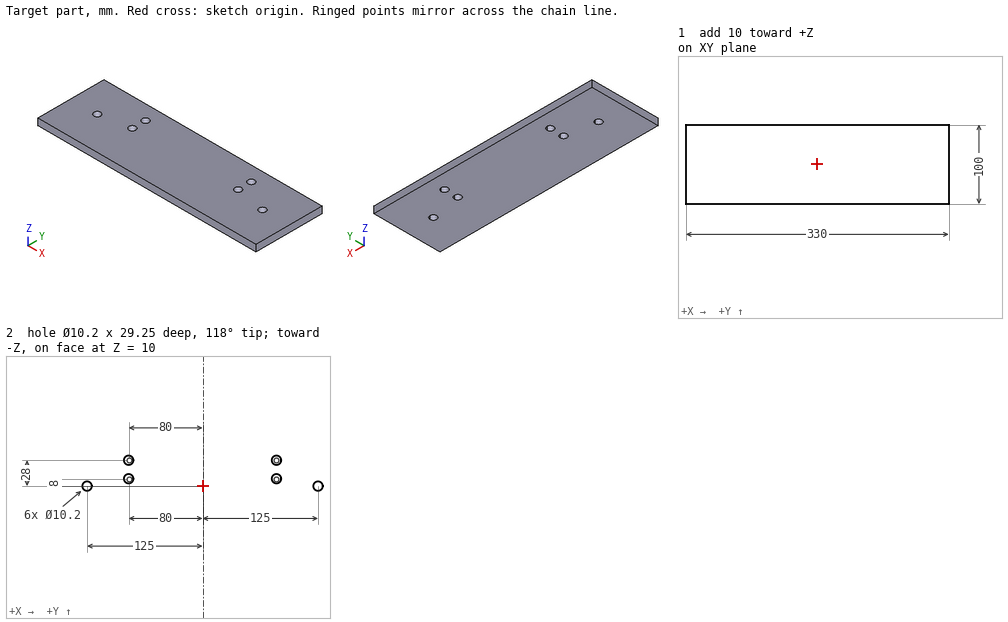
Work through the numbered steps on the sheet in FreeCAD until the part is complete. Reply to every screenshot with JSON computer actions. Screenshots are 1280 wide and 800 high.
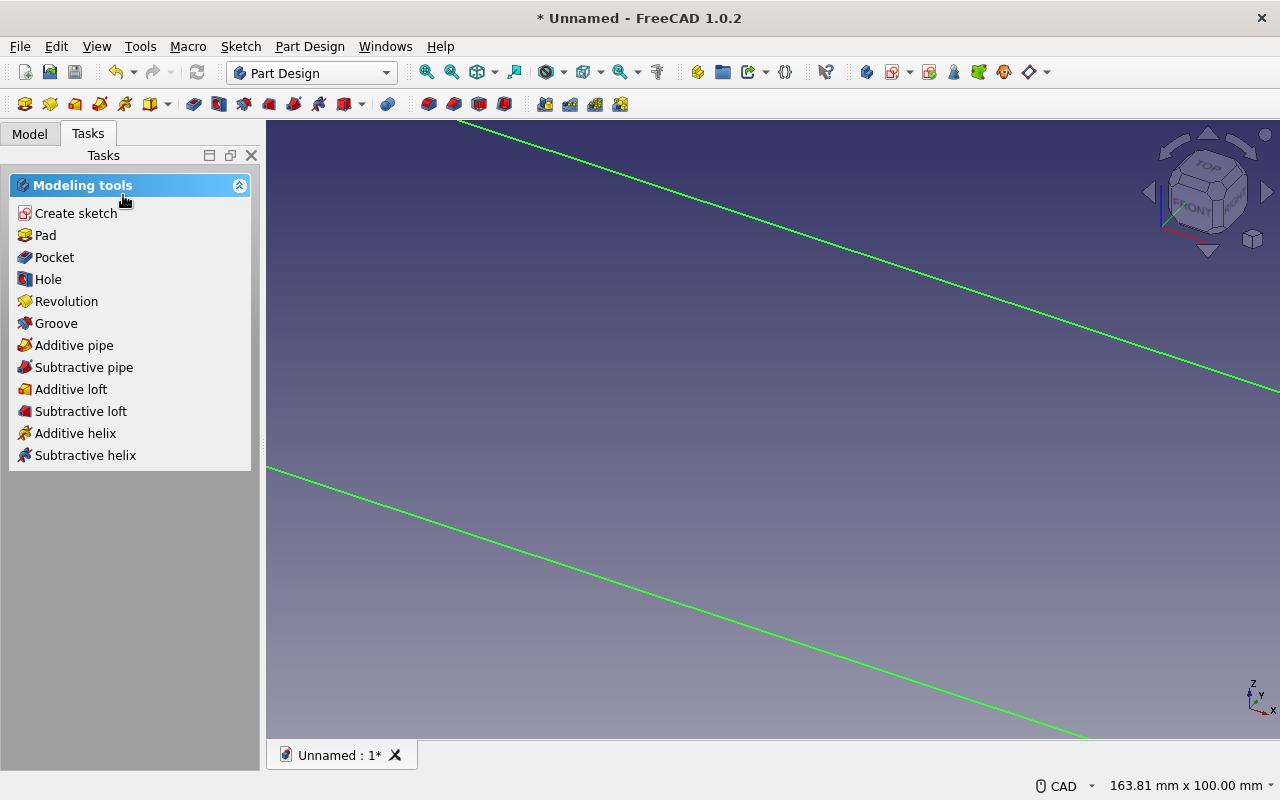
{"action": "left_click", "coordinate": [25, 104]}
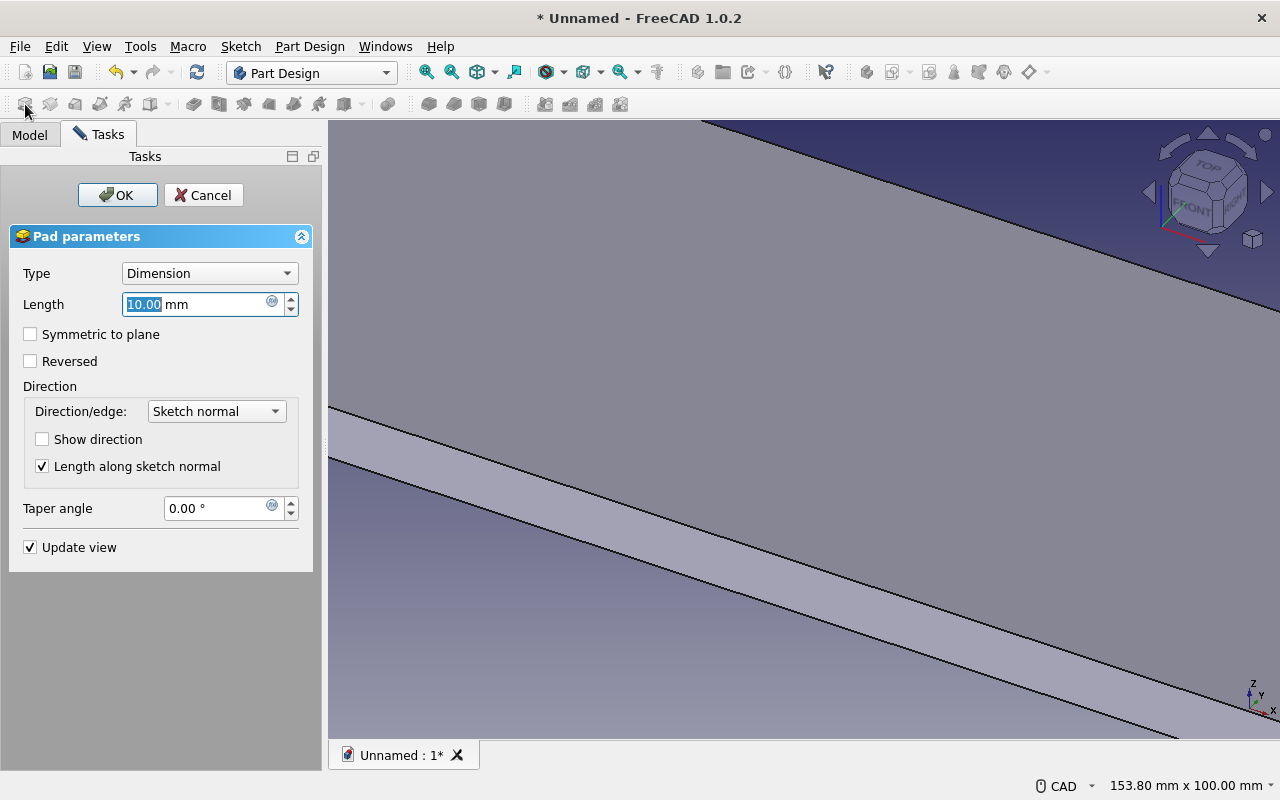
{"action": "type", "text": "10"}
{"action": "key", "text": "Tab"}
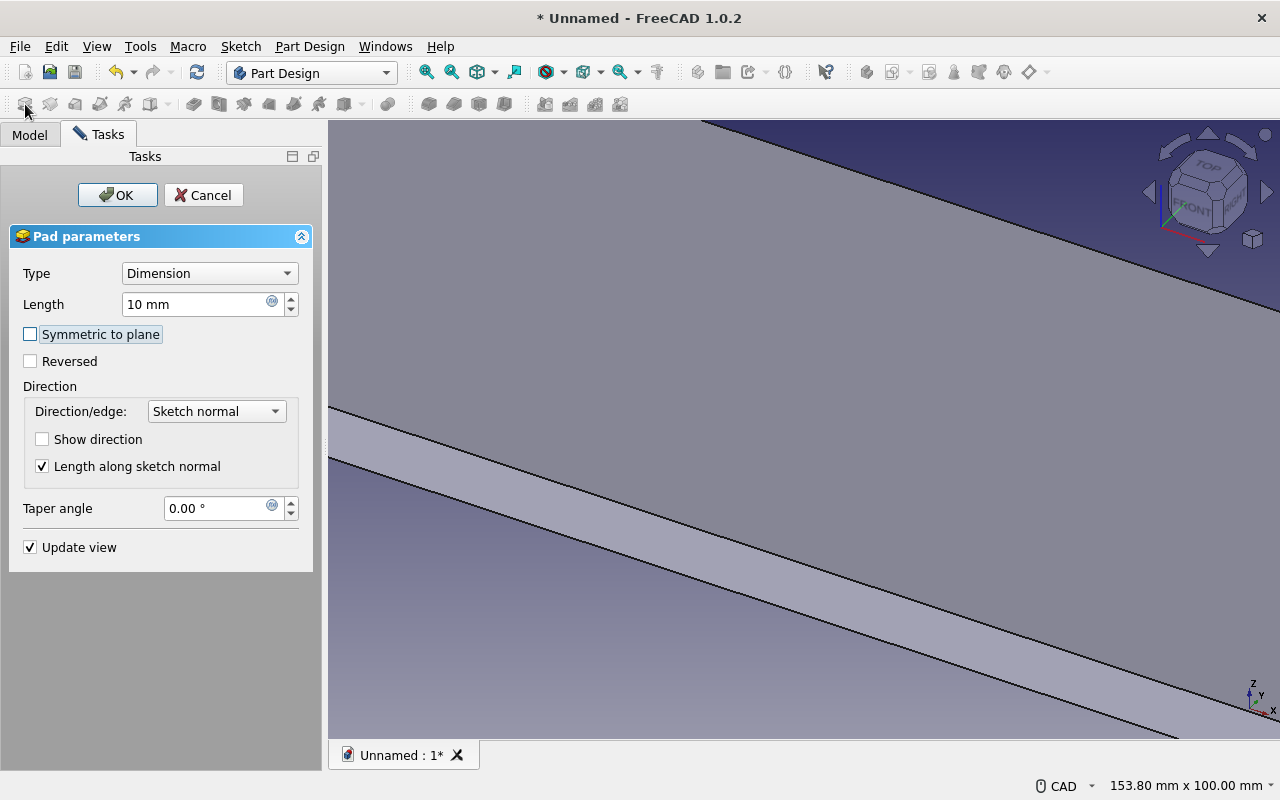
{"action": "left_click", "coordinate": [118, 195]}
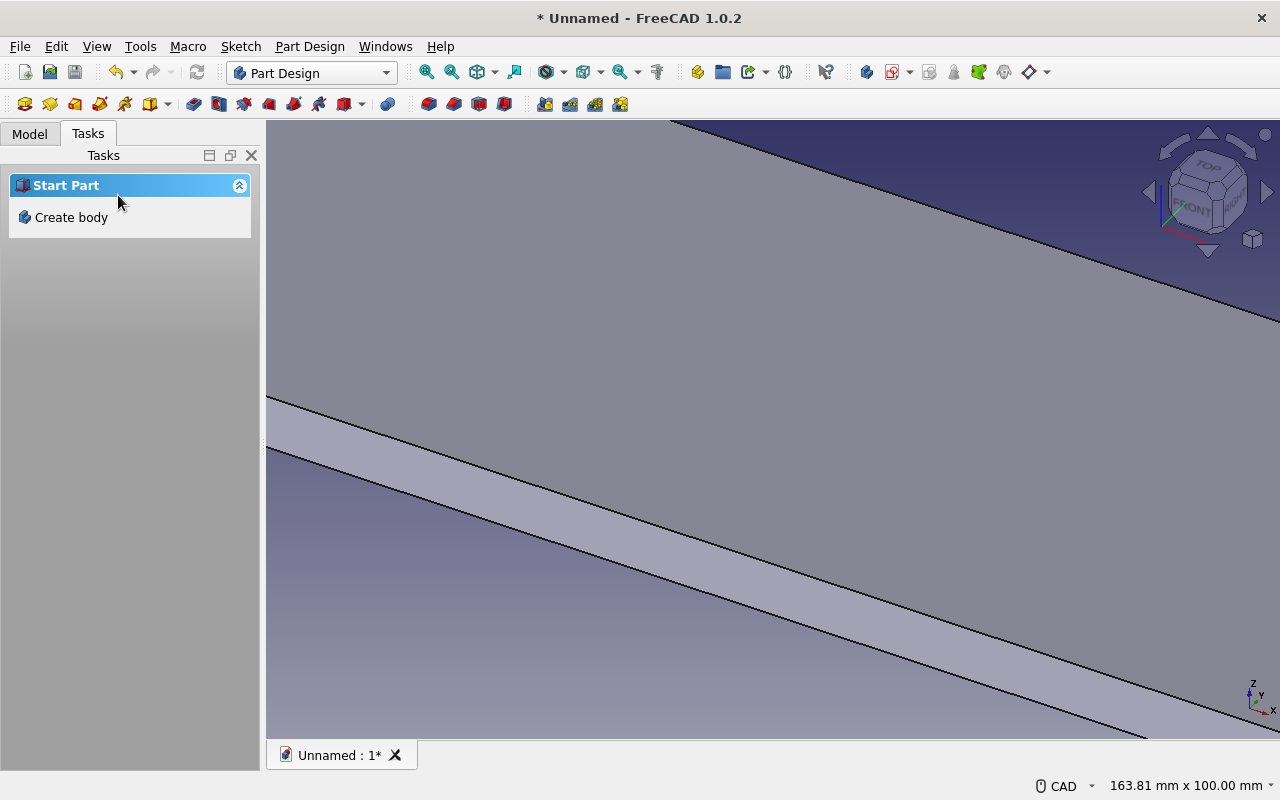
{"action": "left_click", "coordinate": [427, 72]}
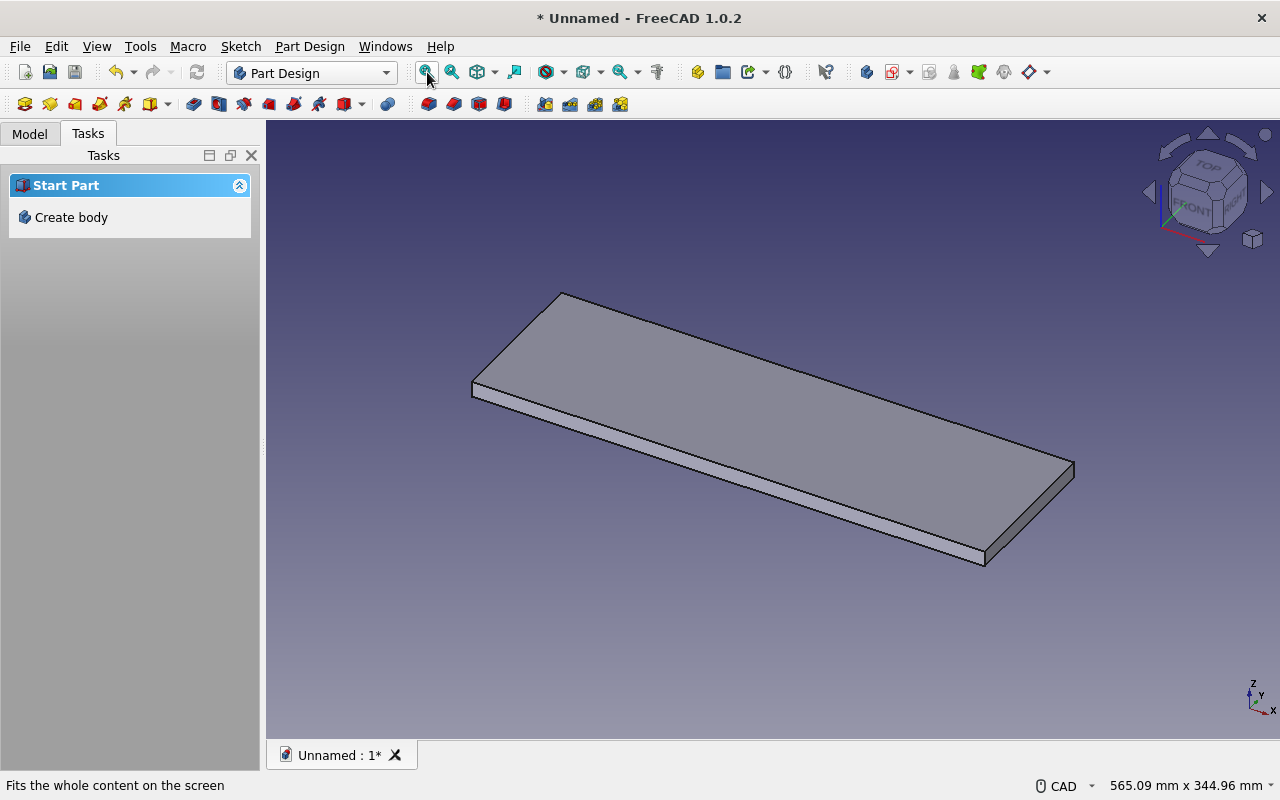
{"action": "left_click", "coordinate": [920, 470]}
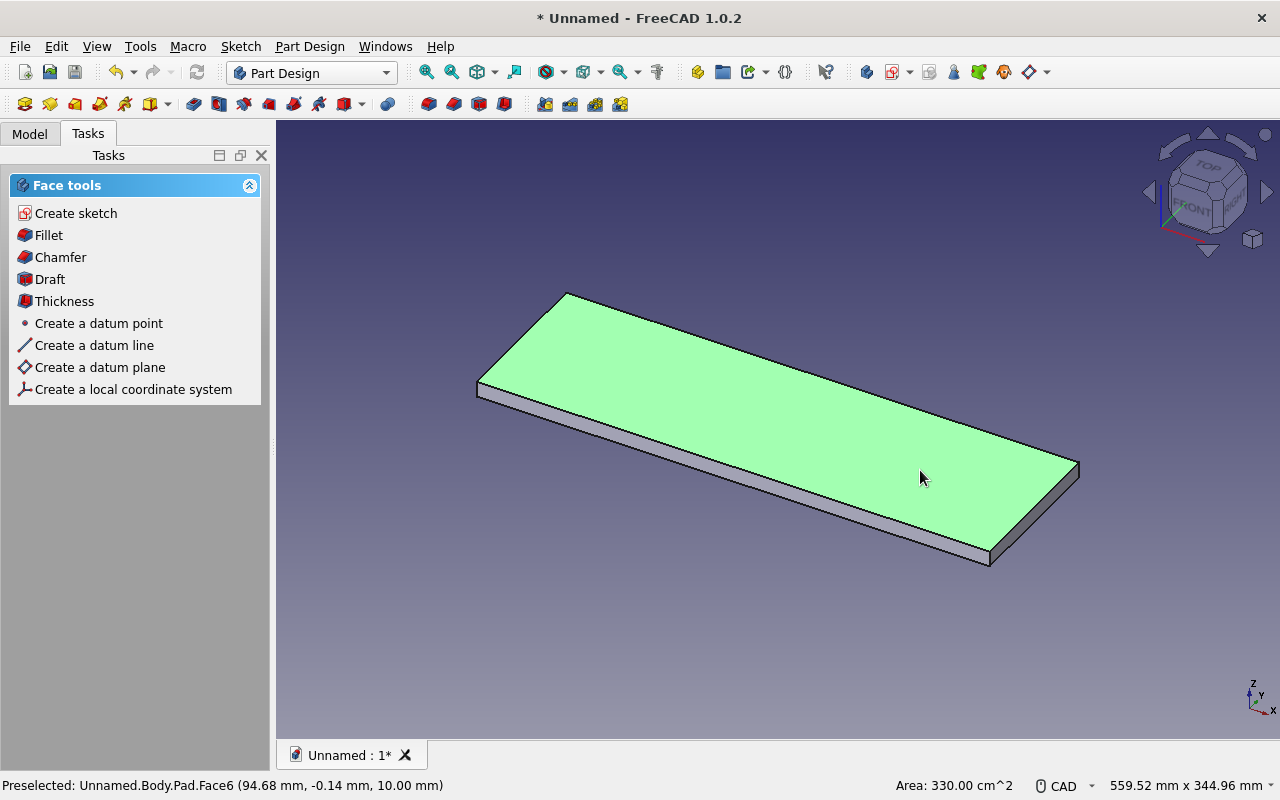
{"action": "left_click", "coordinate": [892, 72]}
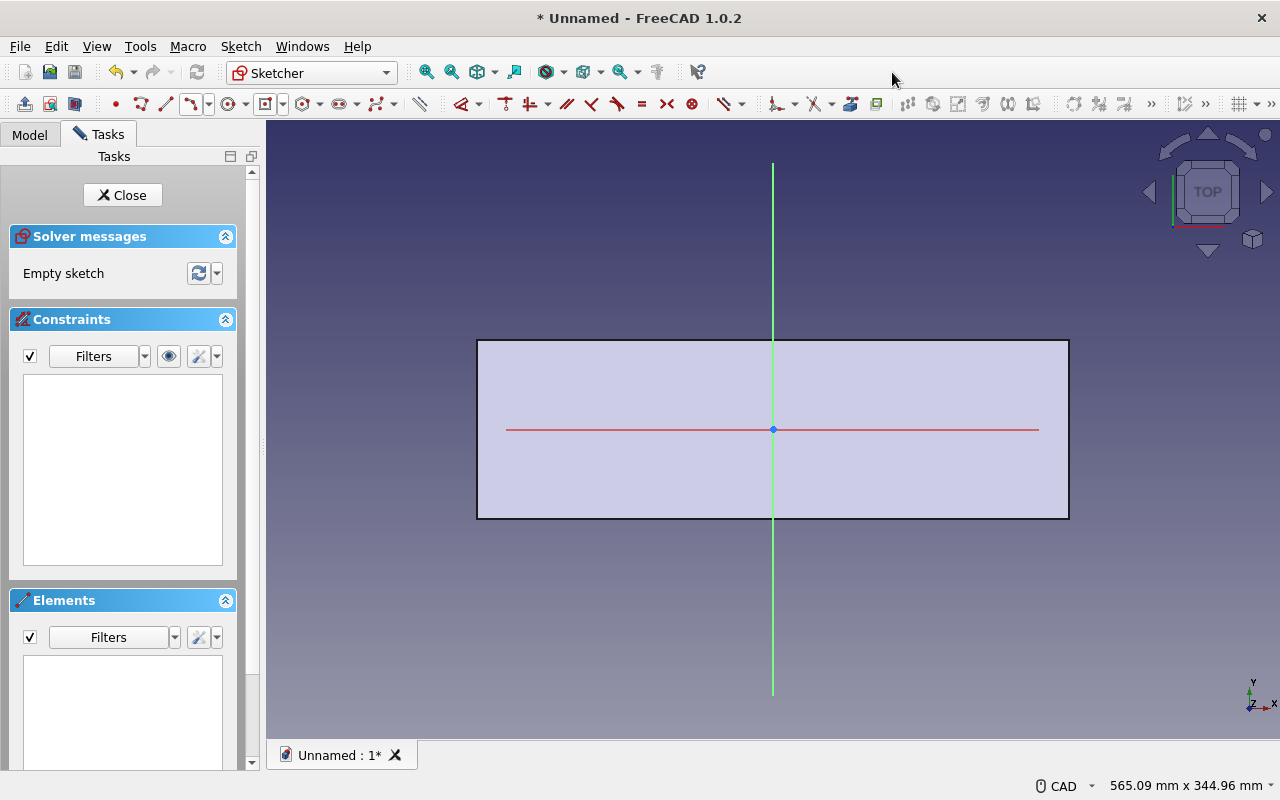
{"action": "left_click", "coordinate": [228, 104]}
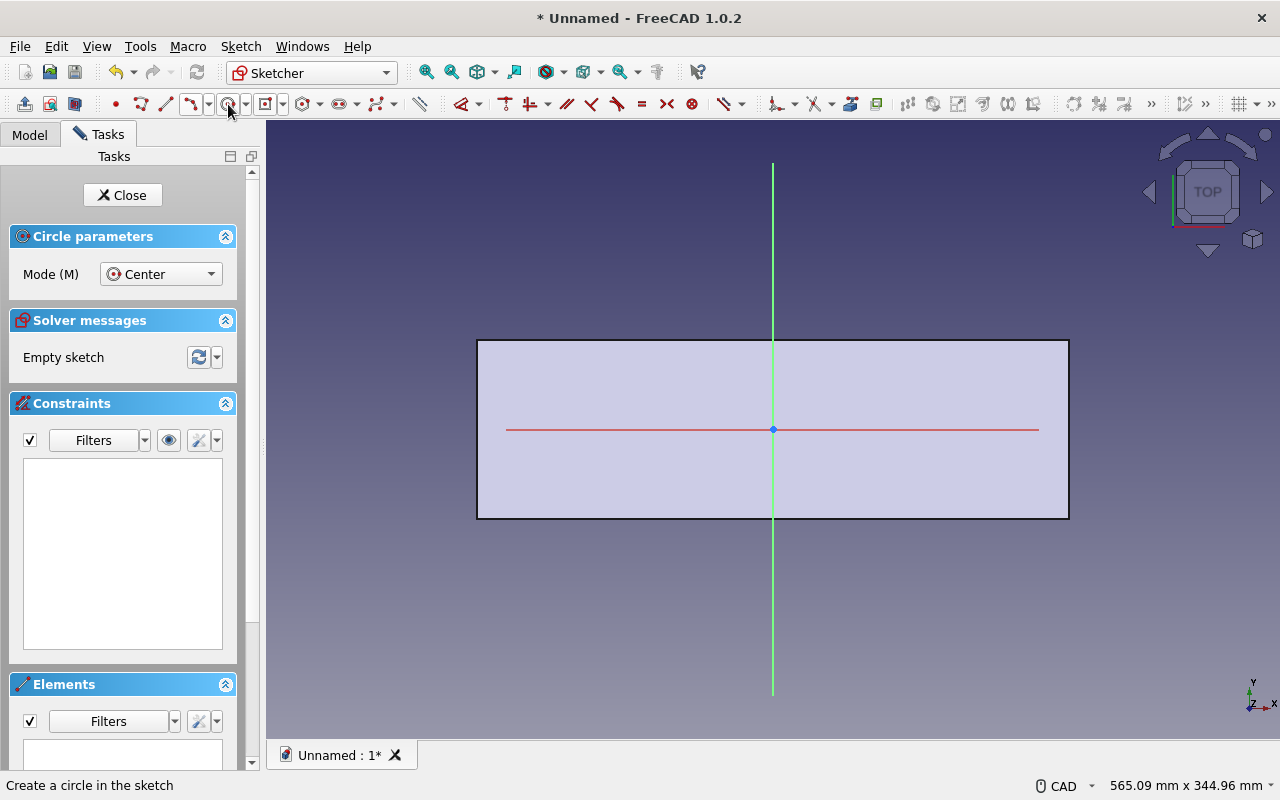
{"action": "scroll", "coordinate": [549, 430], "scroll_direction": "up", "scroll_amount": 5}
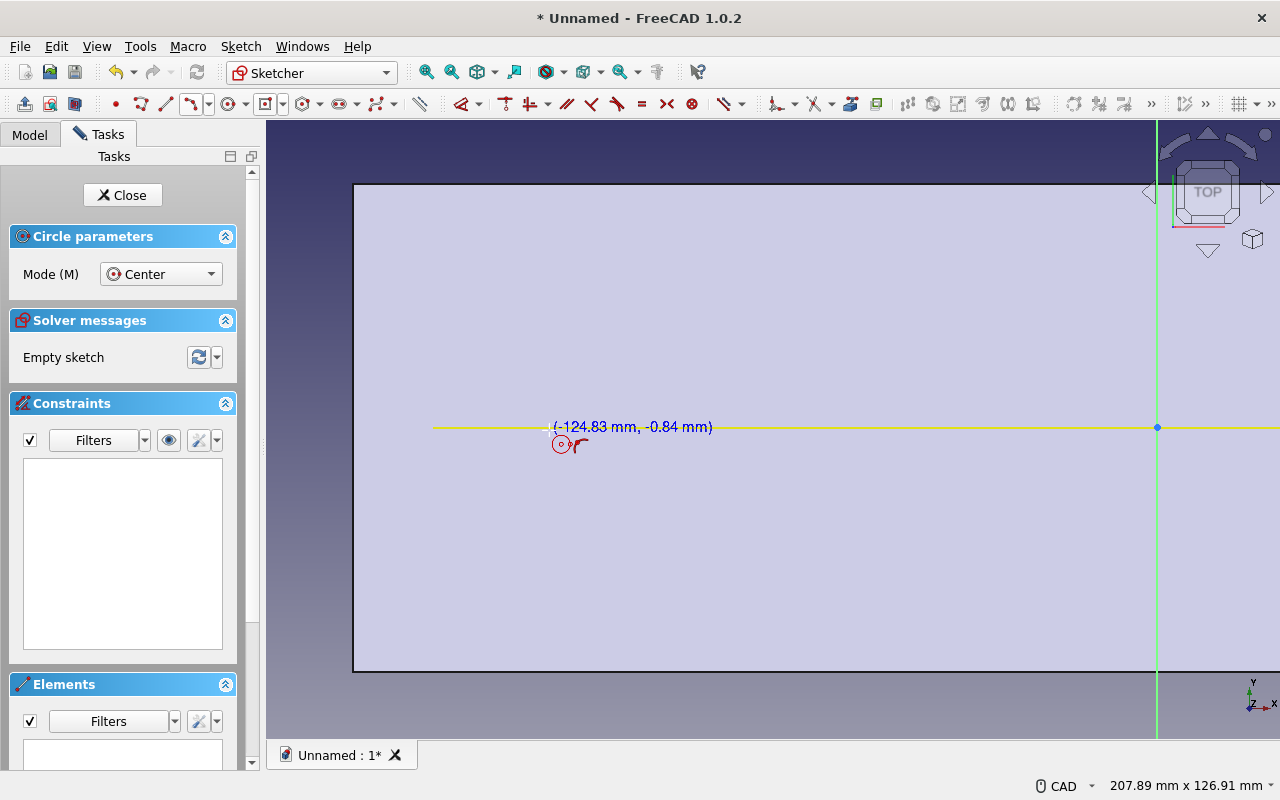
{"action": "left_click", "coordinate": [548, 428]}
{"action": "mouse_move", "coordinate": [565, 410]}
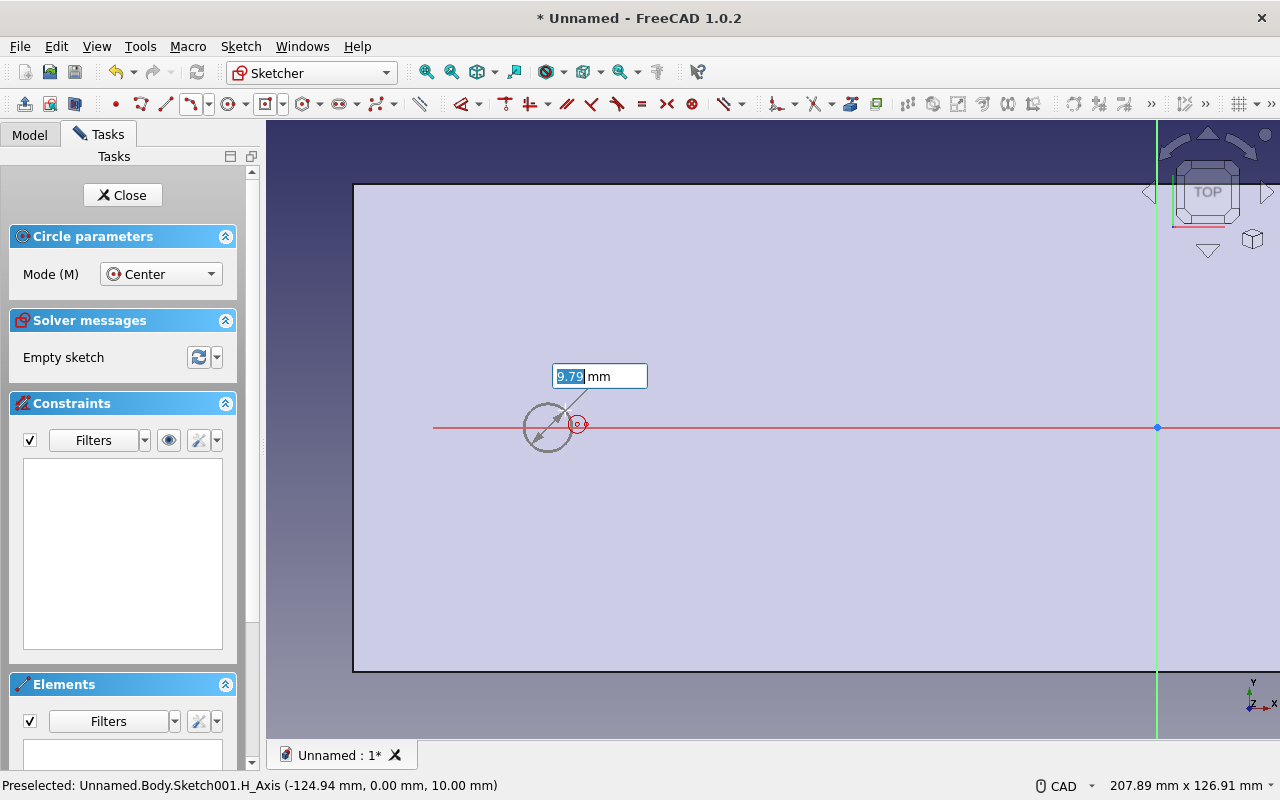
{"action": "type", "text": "10.2"}
{"action": "key", "text": "Return"}